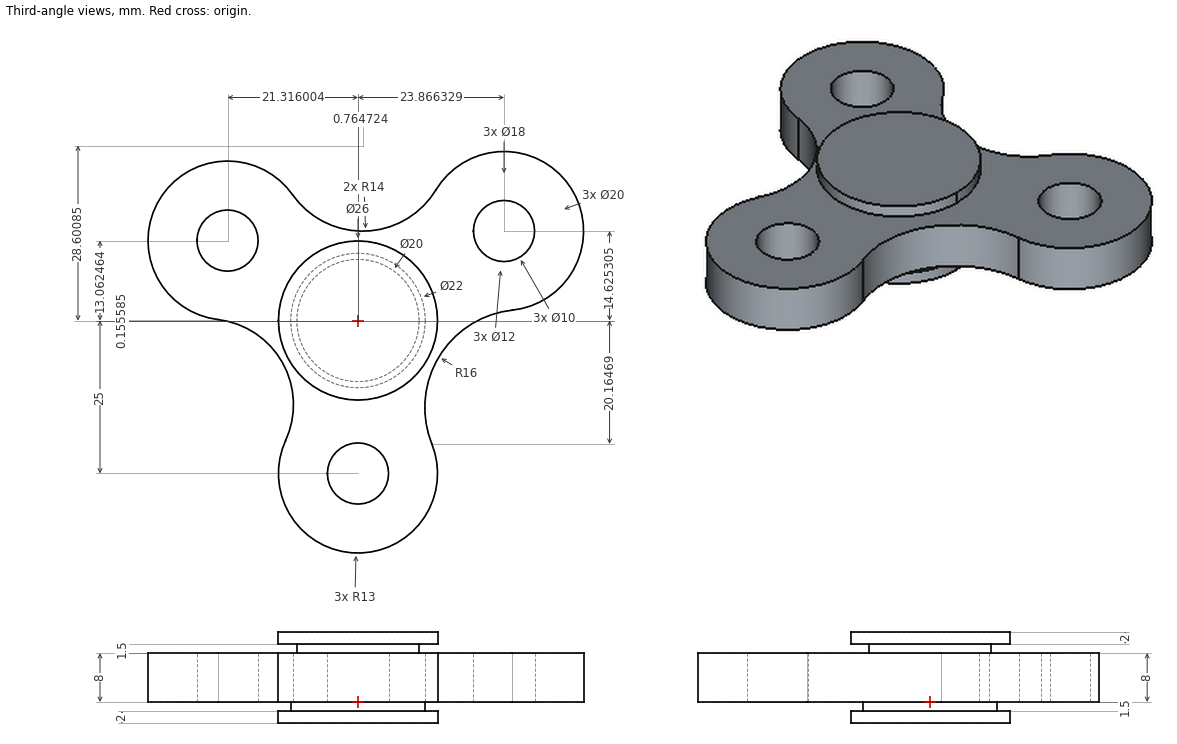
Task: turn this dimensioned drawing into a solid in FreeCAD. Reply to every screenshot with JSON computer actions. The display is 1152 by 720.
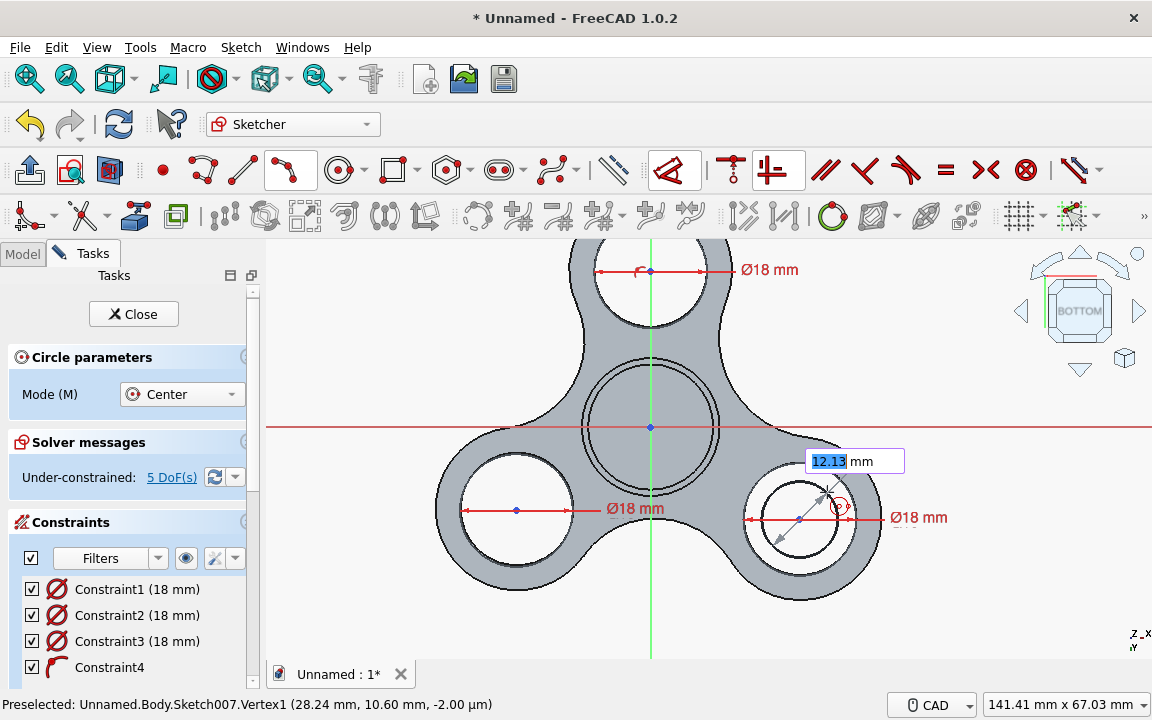
{"action": "type", "text": "12"}
{"action": "key", "text": "Return"}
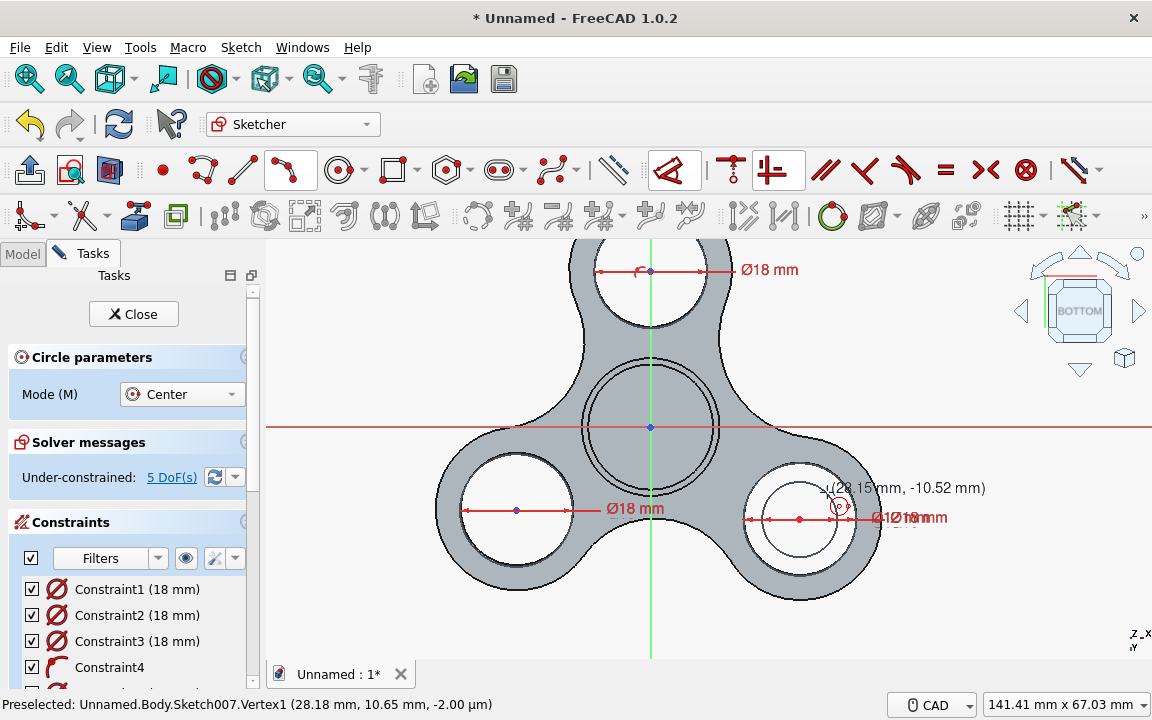
{"action": "left_click", "coordinate": [516, 511]}
{"action": "mouse_move", "coordinate": [544, 482]}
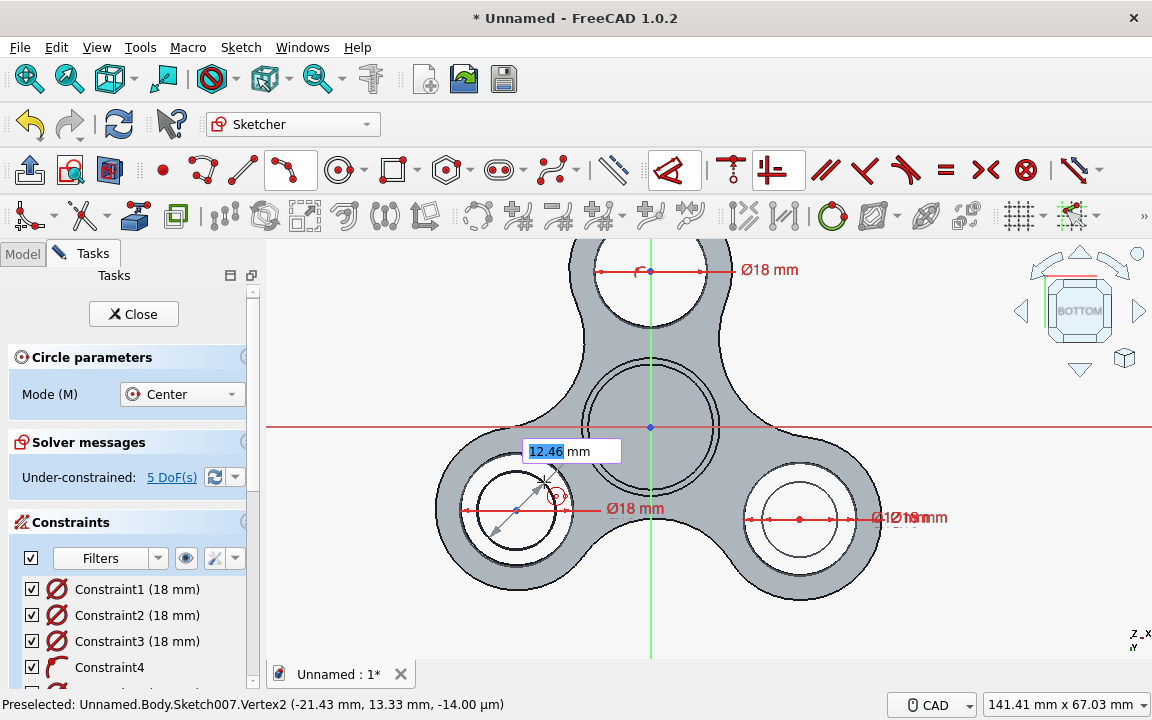
{"action": "type", "text": "12"}
{"action": "key", "text": "Return"}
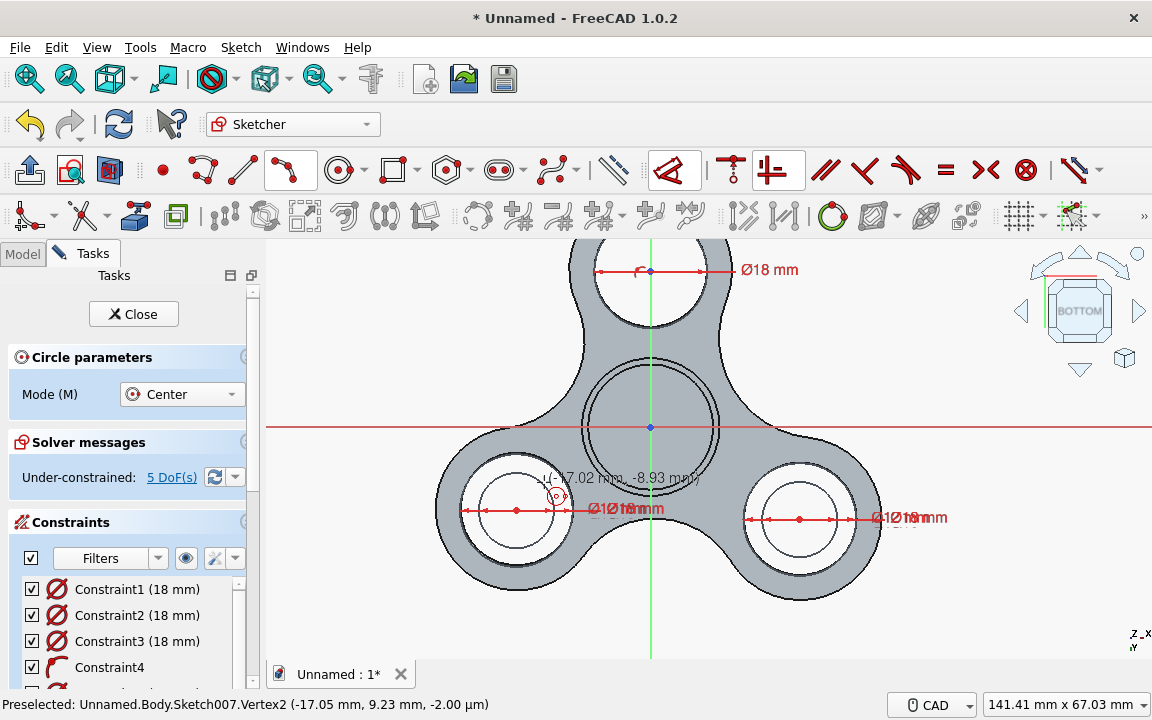
{"action": "left_click", "coordinate": [651, 272]}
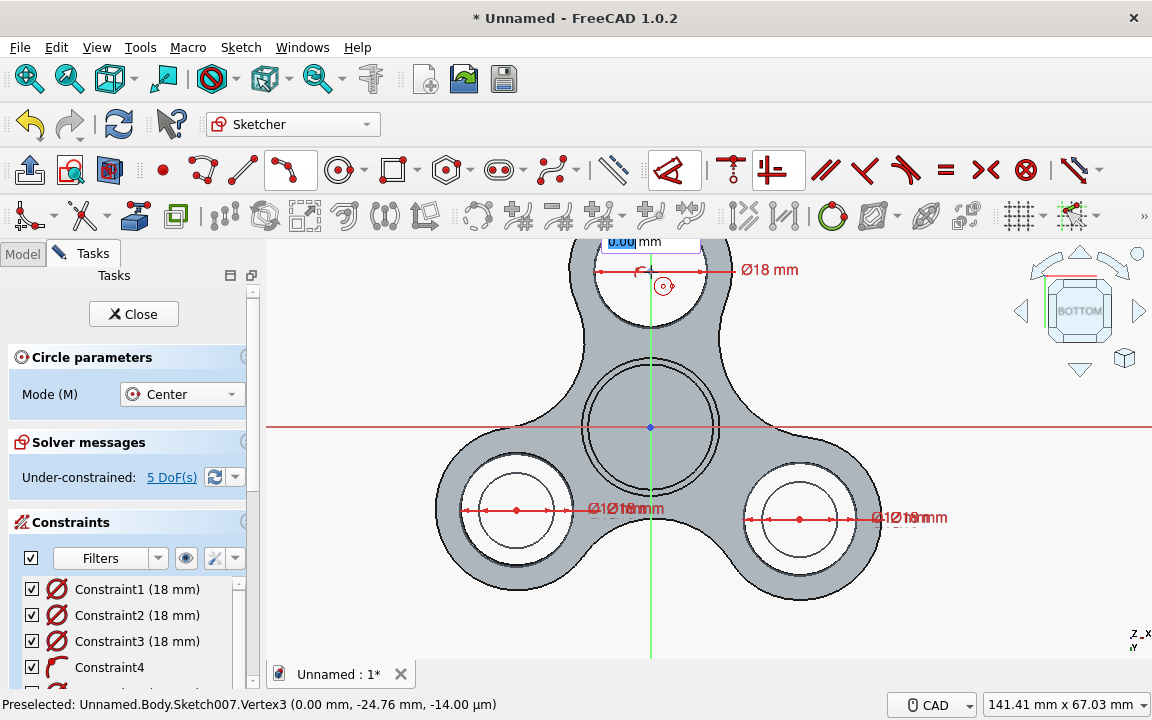
{"action": "scroll", "coordinate": [604, 560], "scroll_direction": "down", "scroll_amount": 2}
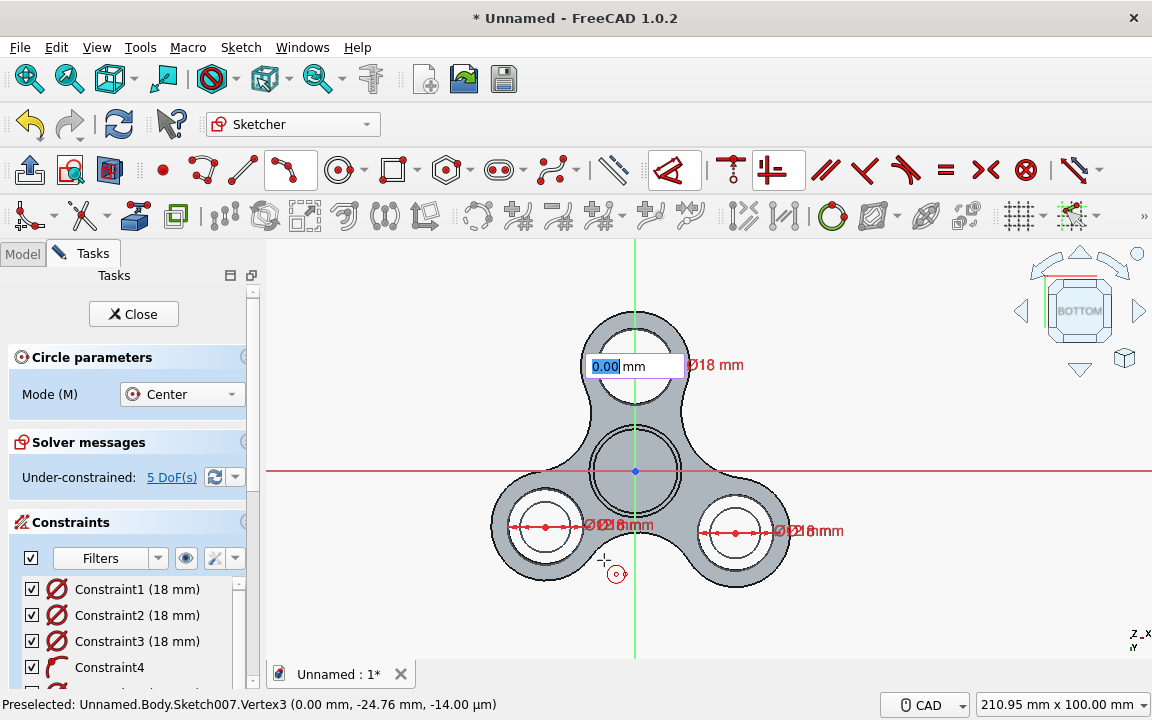
{"action": "scroll", "coordinate": [653, 348], "scroll_direction": "up", "scroll_amount": 2}
{"action": "mouse_move", "coordinate": [653, 348]}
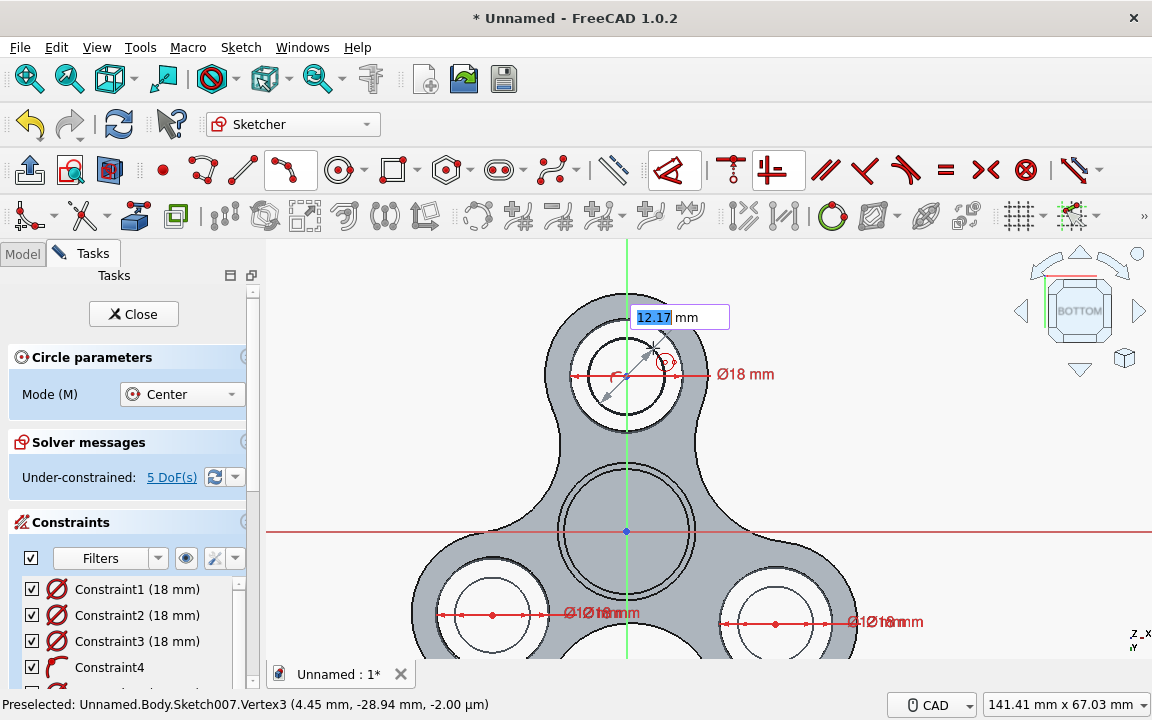
{"action": "type", "text": "12"}
{"action": "key", "text": "Return"}
{"action": "key", "text": "Escape"}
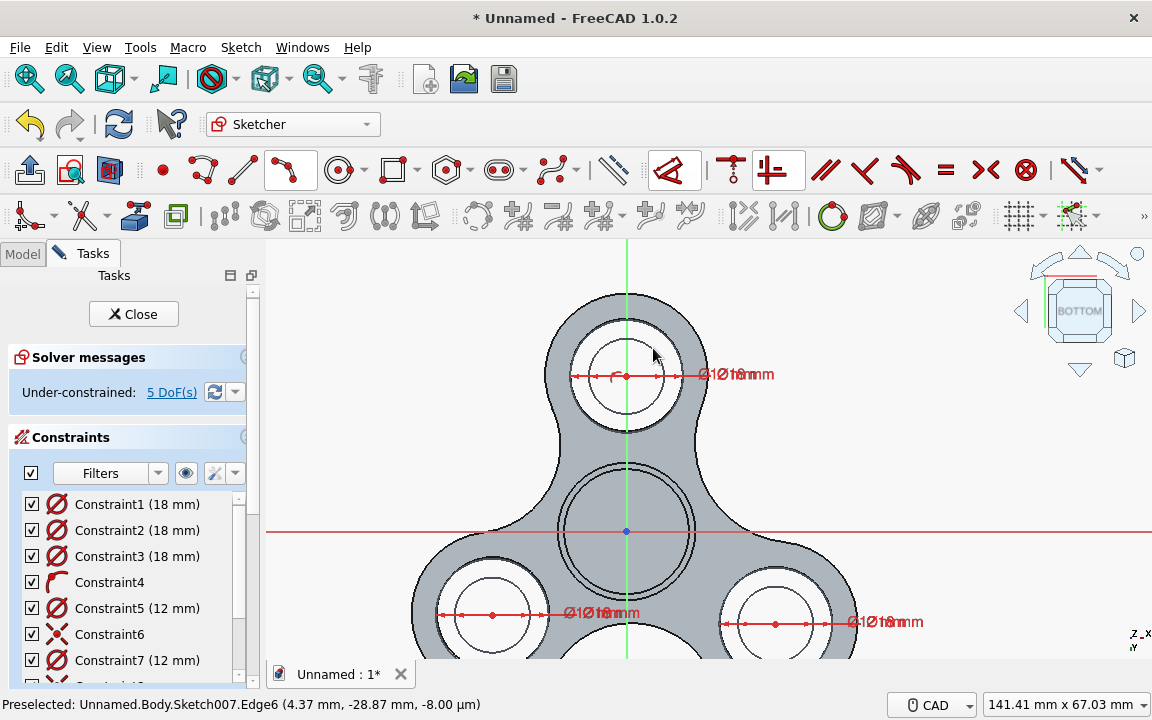
{"action": "left_click", "coordinate": [627, 376]}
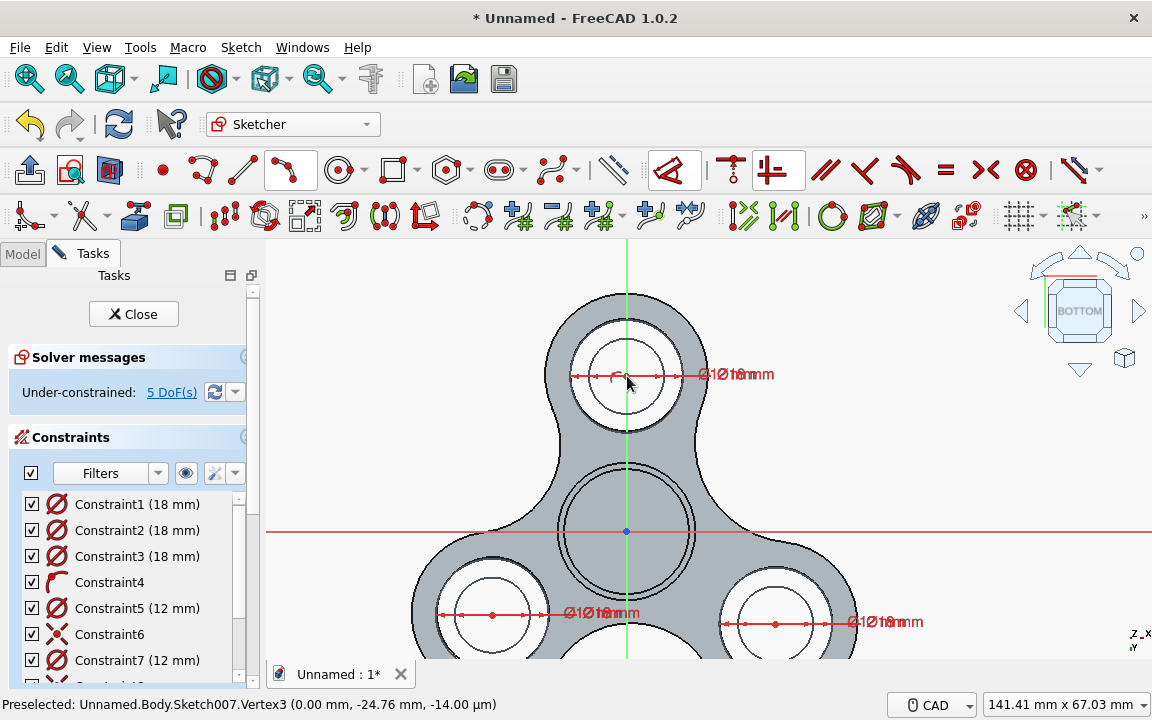
{"action": "left_click", "coordinate": [696, 170]}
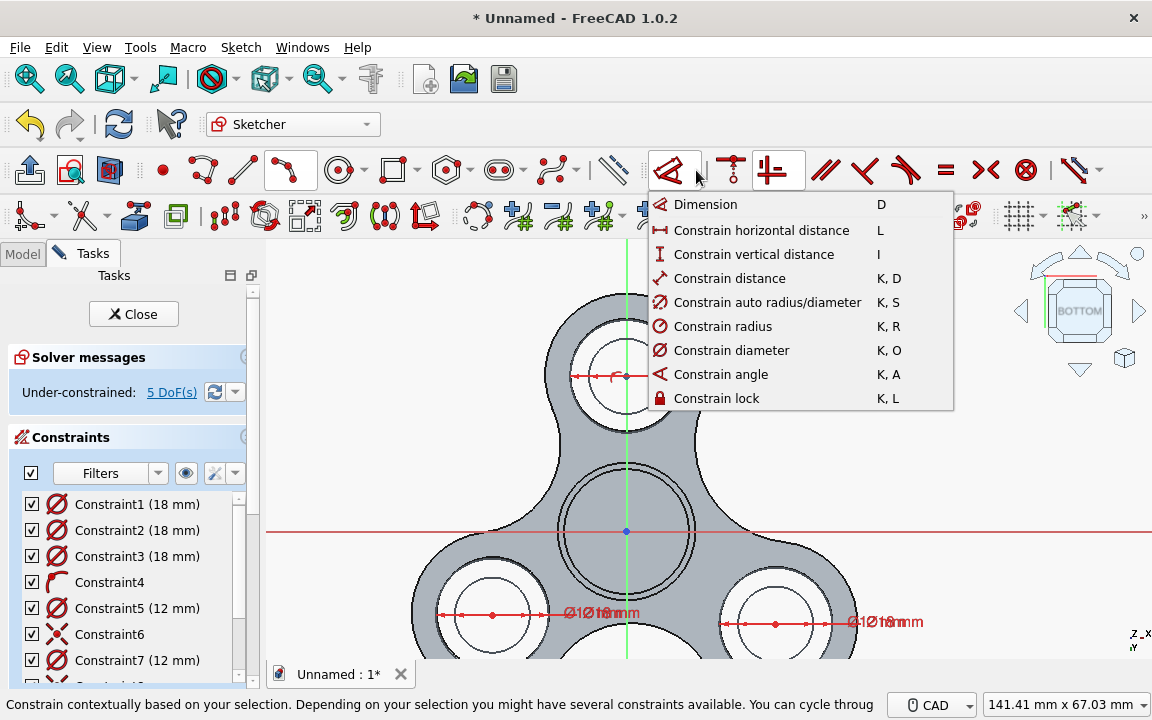
{"action": "left_click", "coordinate": [801, 254]}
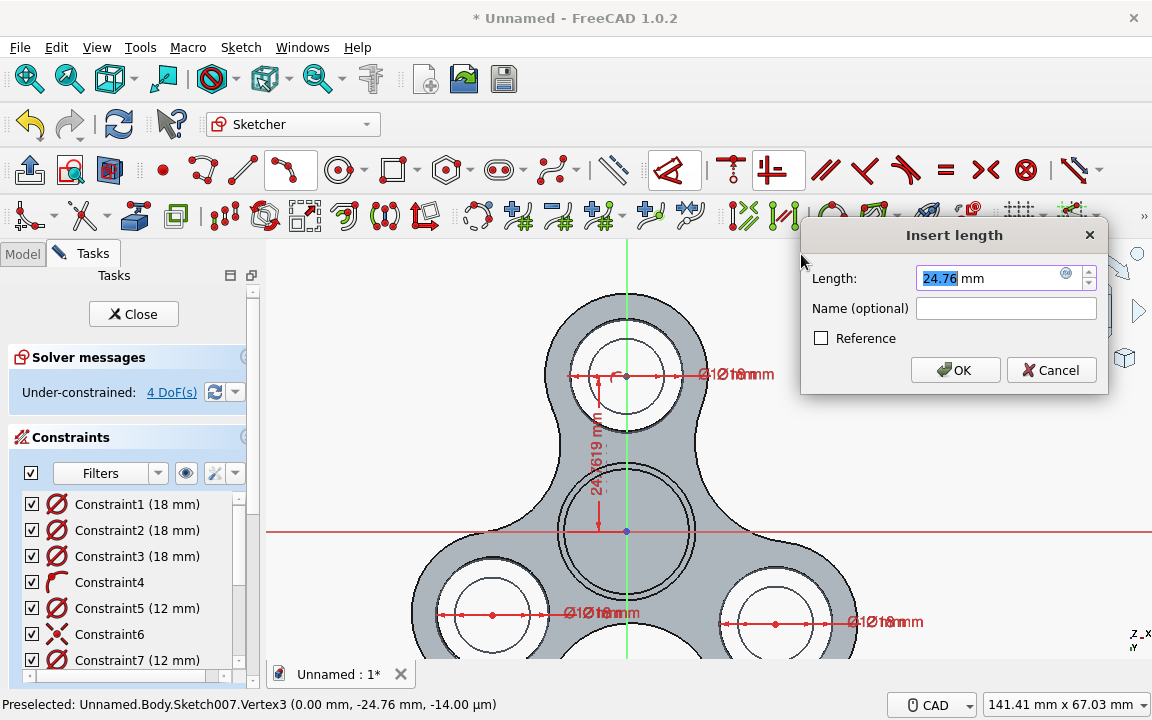
{"action": "type", "text": "25"}
{"action": "key", "text": "Return"}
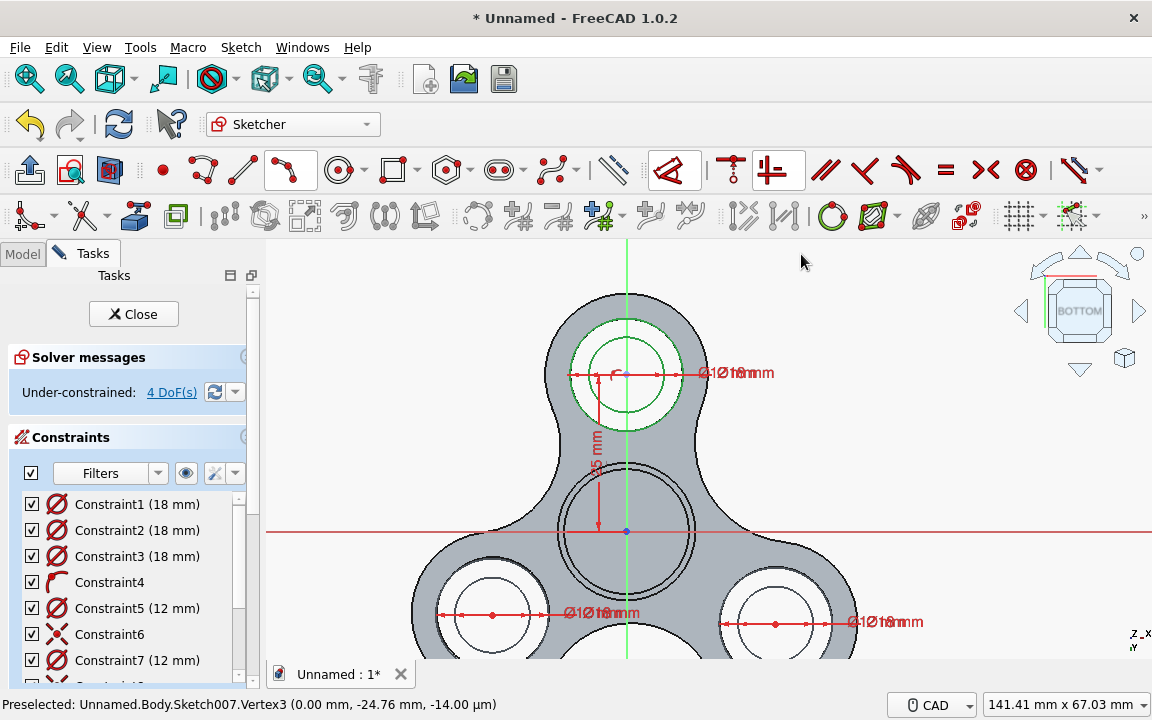
{"action": "left_click", "coordinate": [776, 624]}